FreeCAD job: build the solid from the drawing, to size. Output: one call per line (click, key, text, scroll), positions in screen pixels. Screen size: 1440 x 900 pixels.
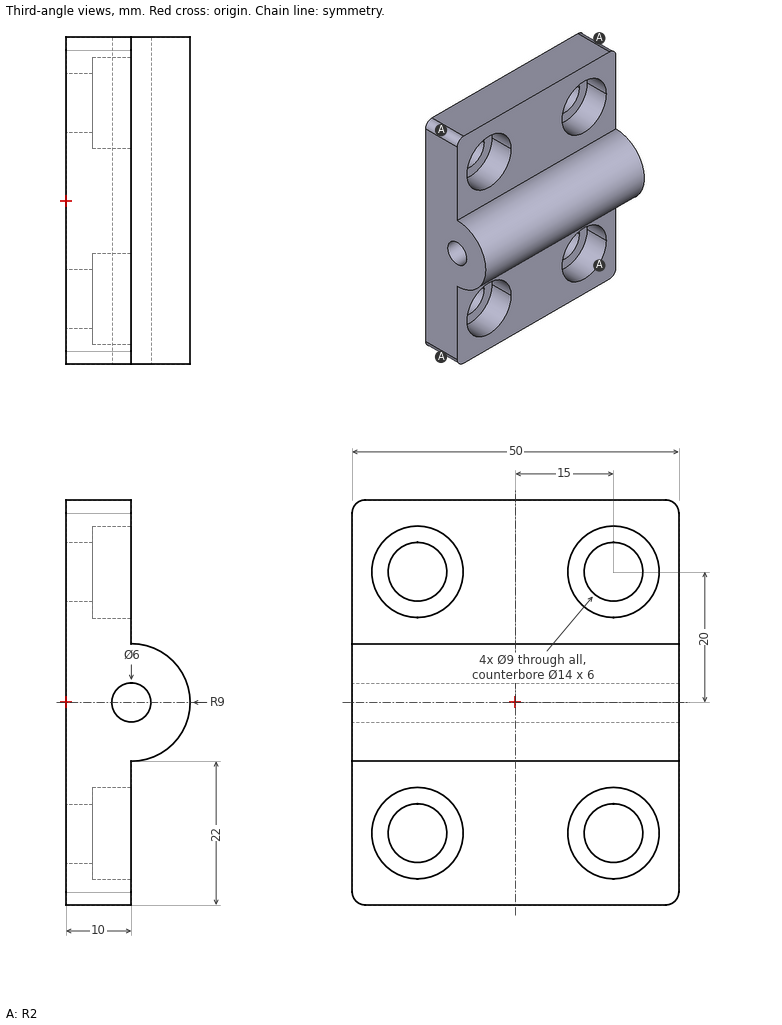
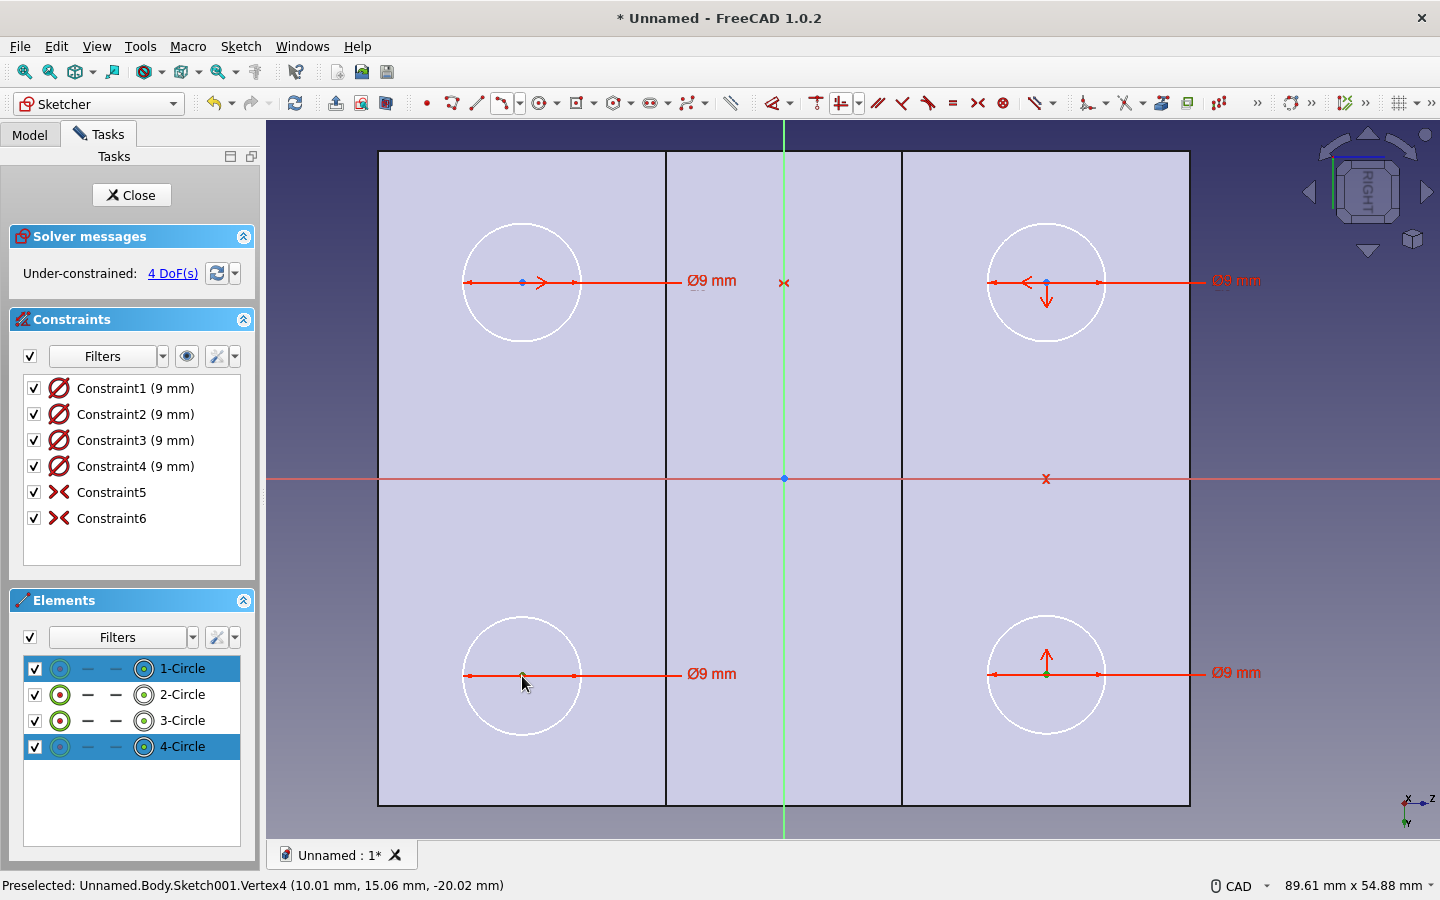
click(784, 764)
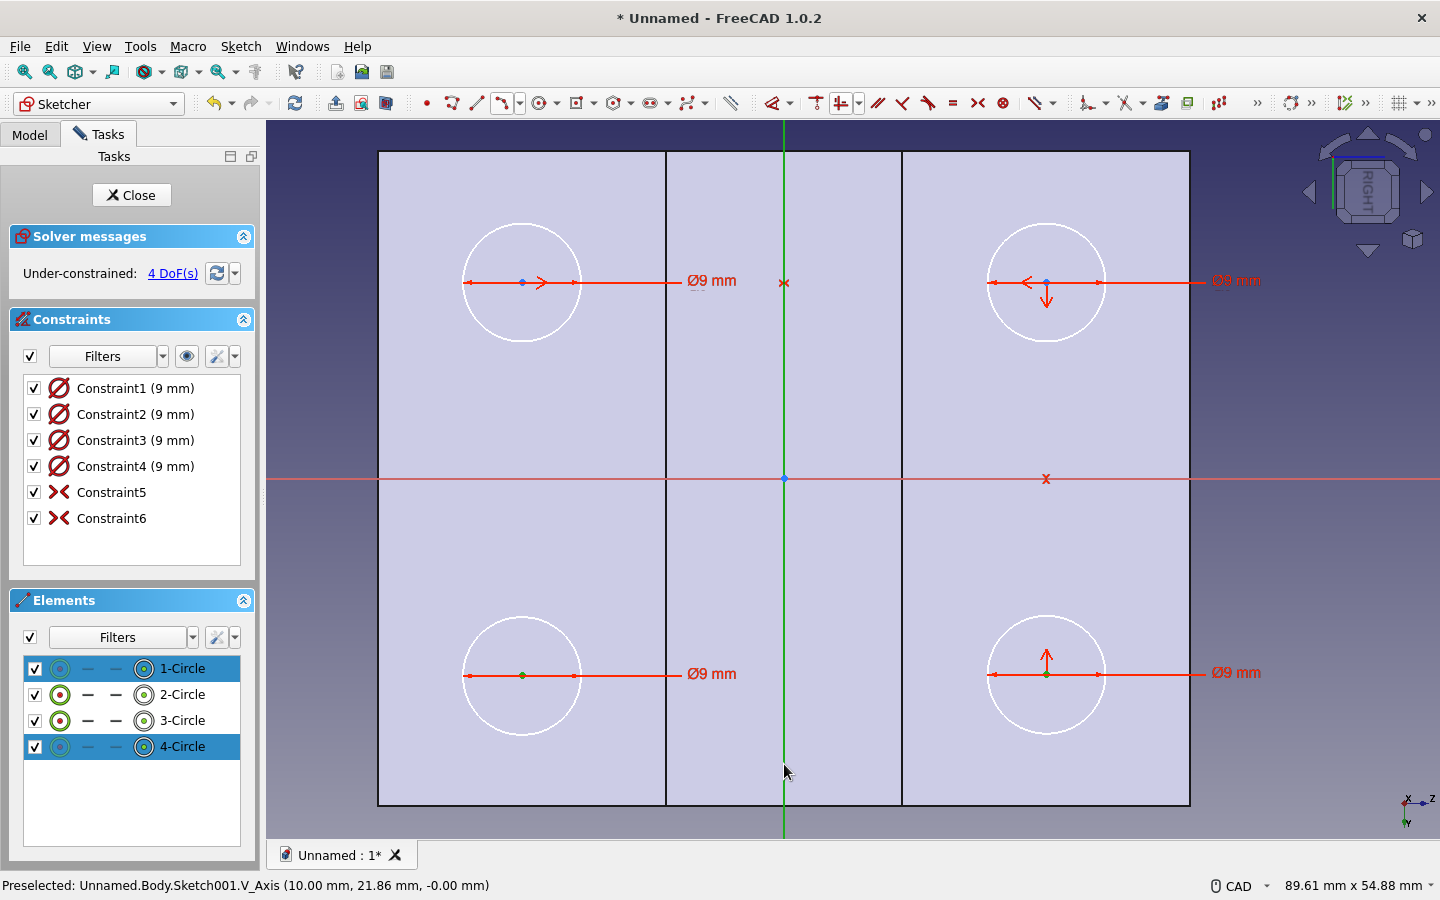
click(978, 104)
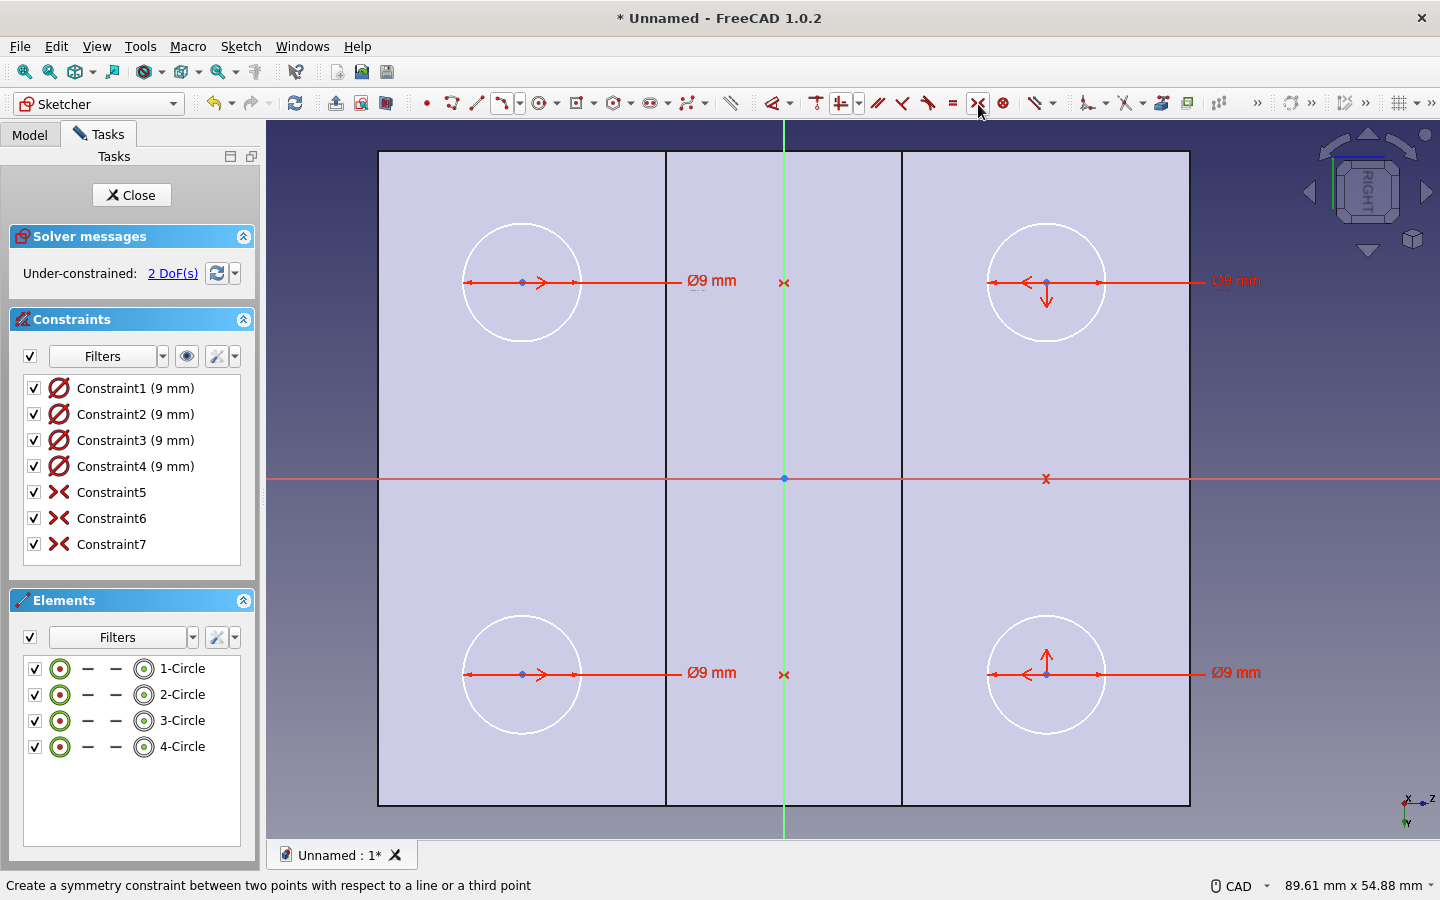
click(772, 104)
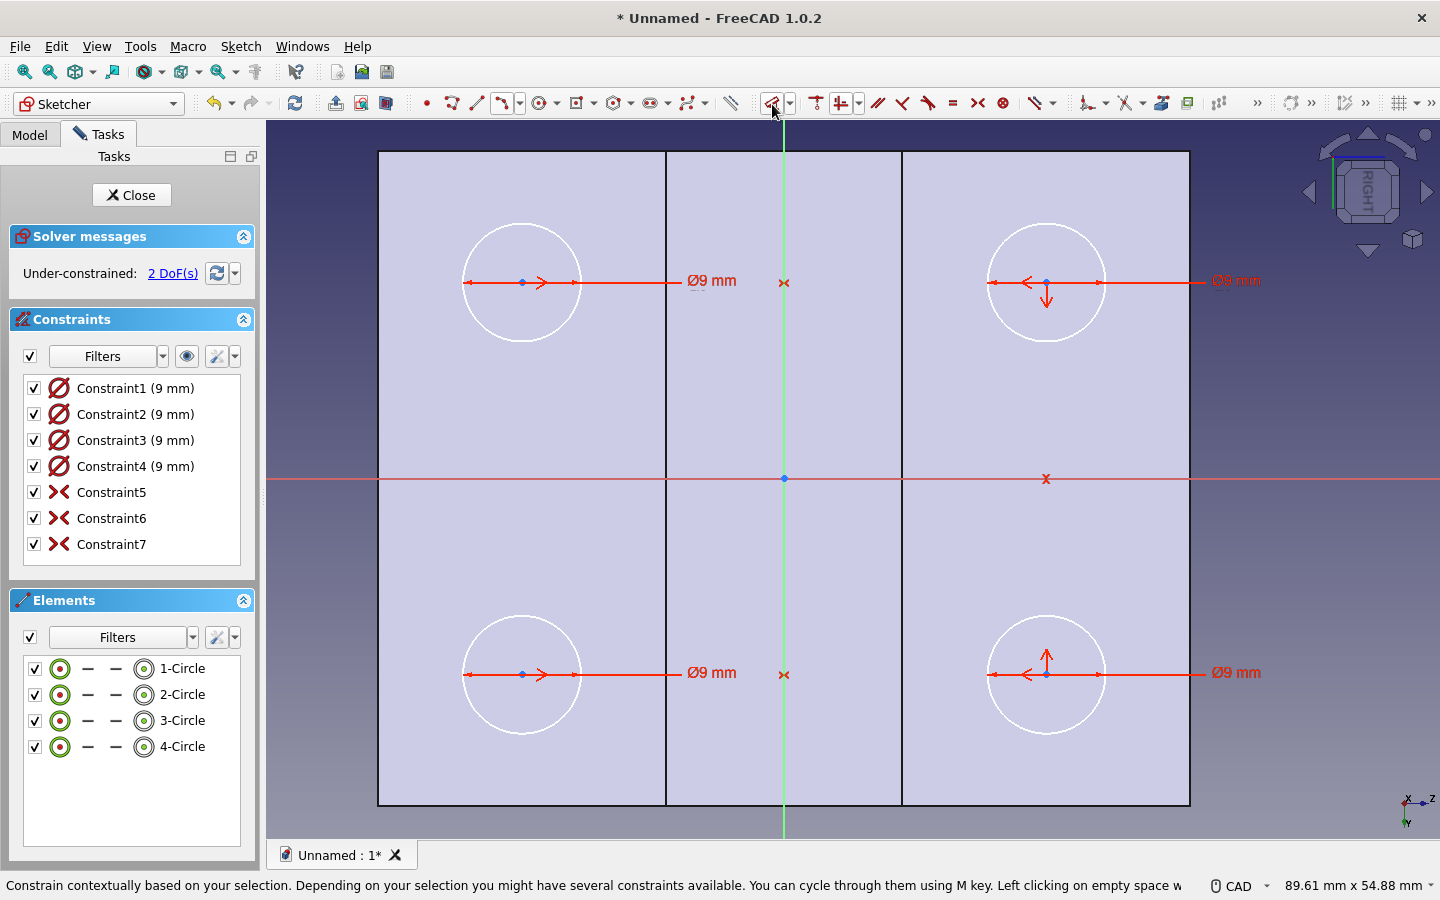
click(1047, 675)
click(915, 709)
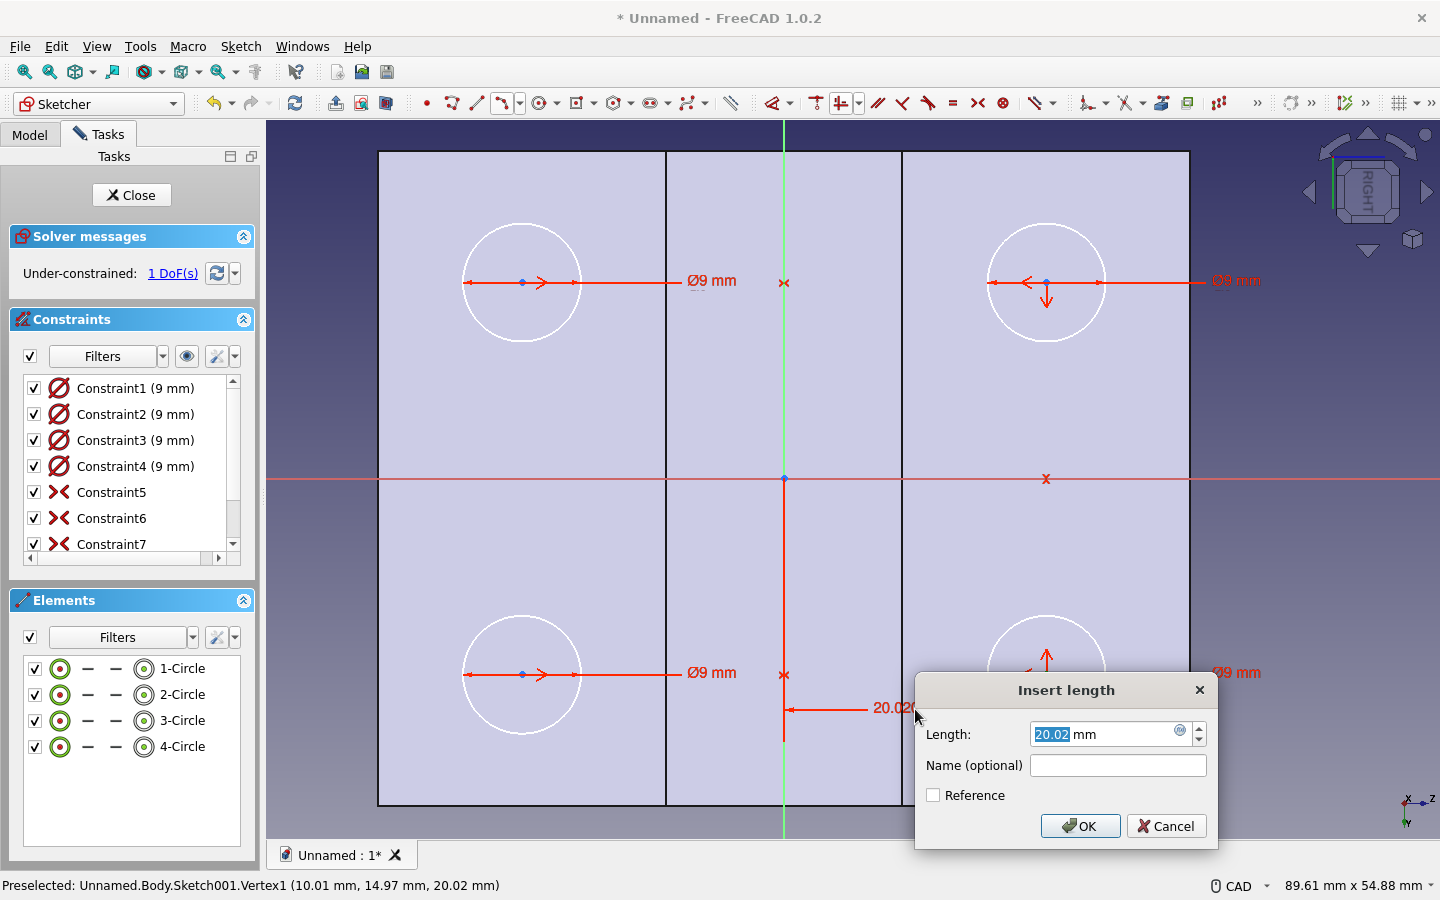
text(20)
key(Return)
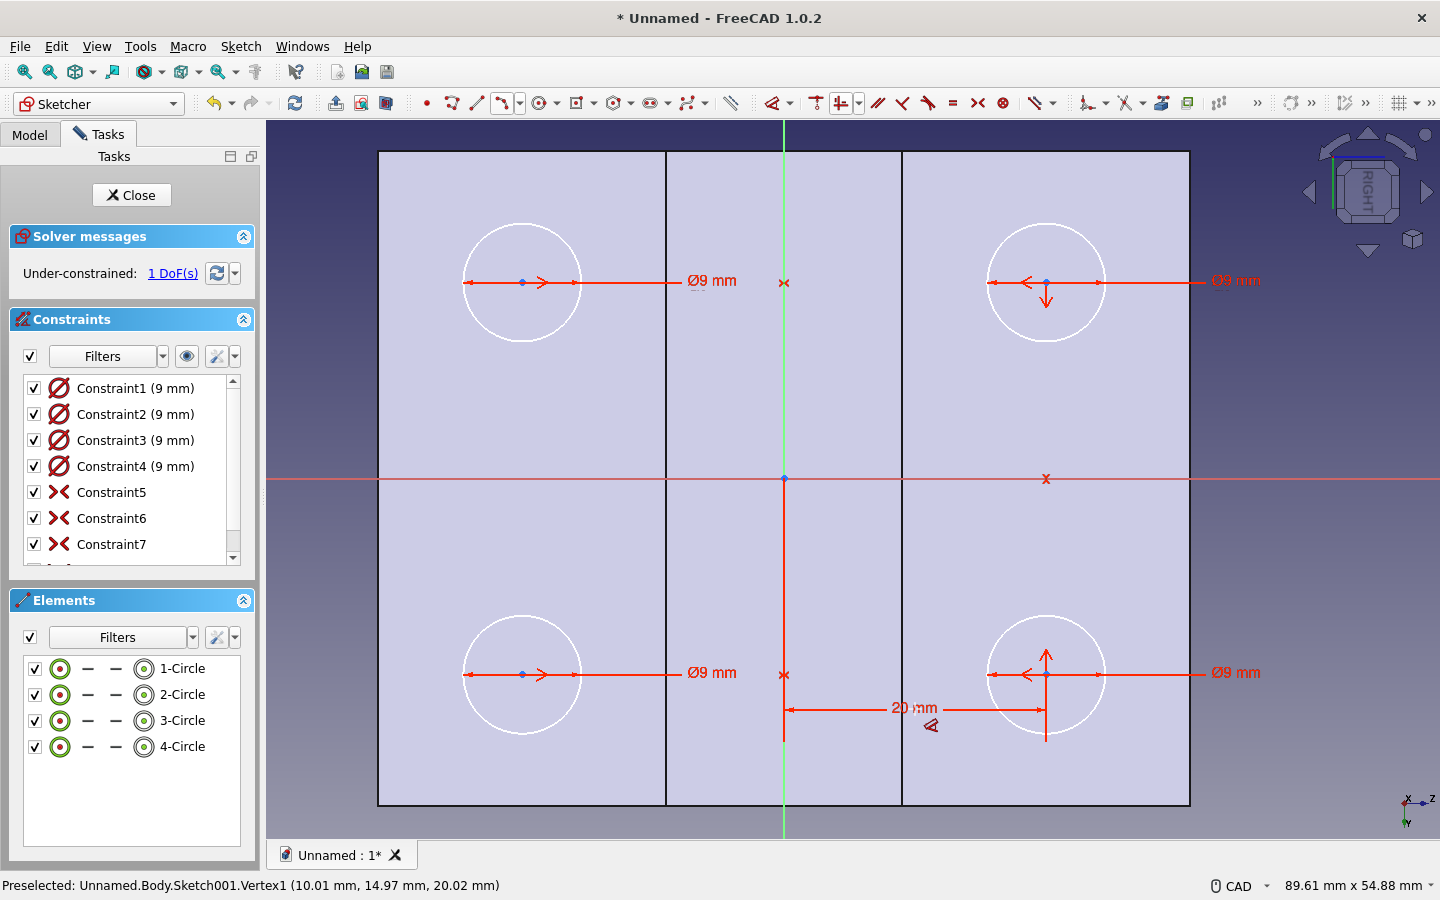
click(1046, 675)
click(1080, 577)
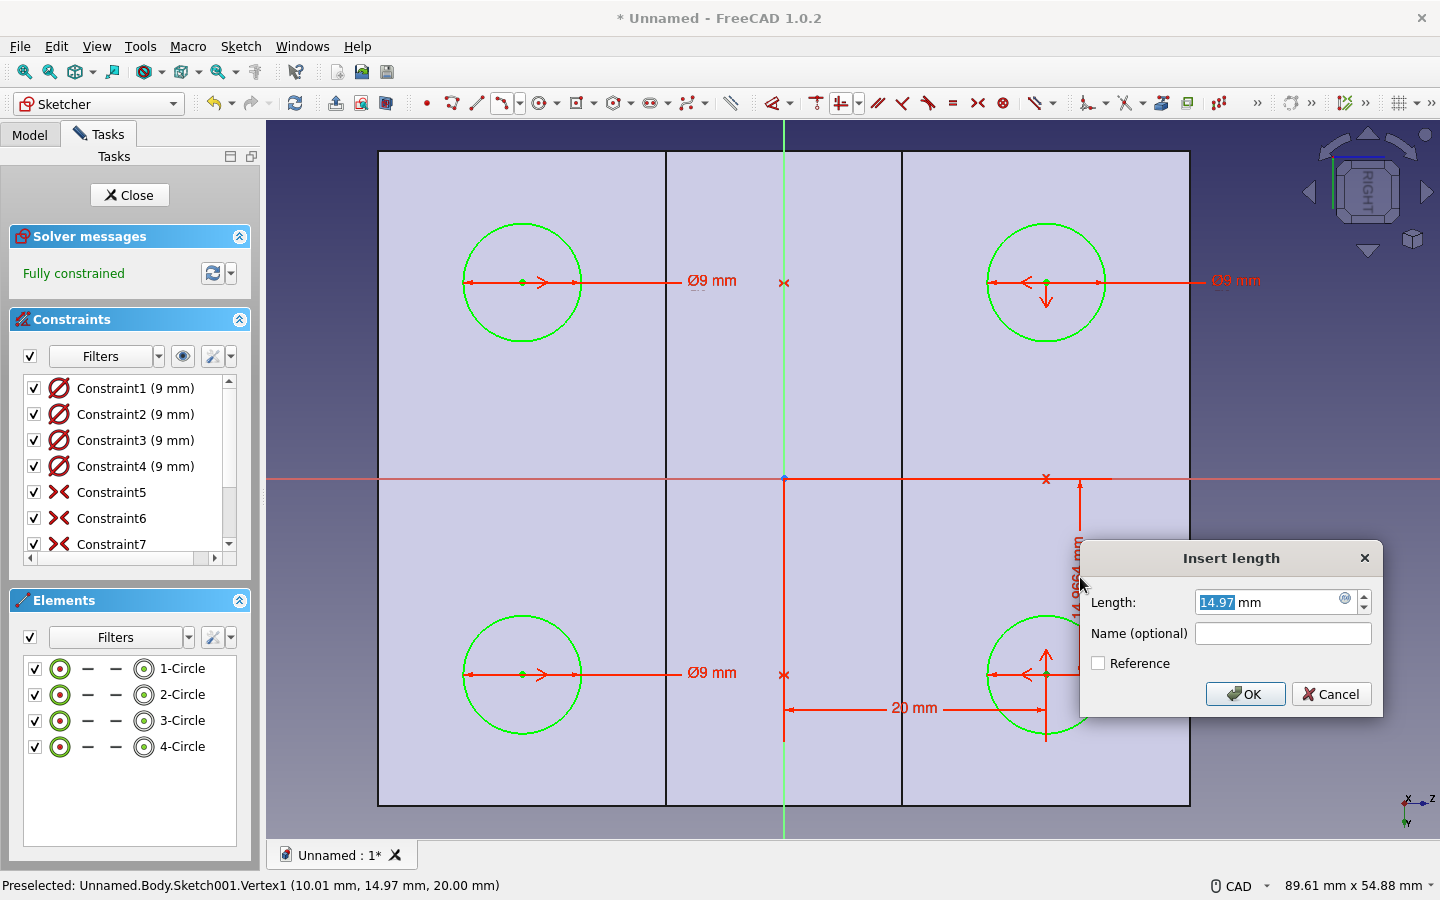
text(15)
key(Return)
key(Escape)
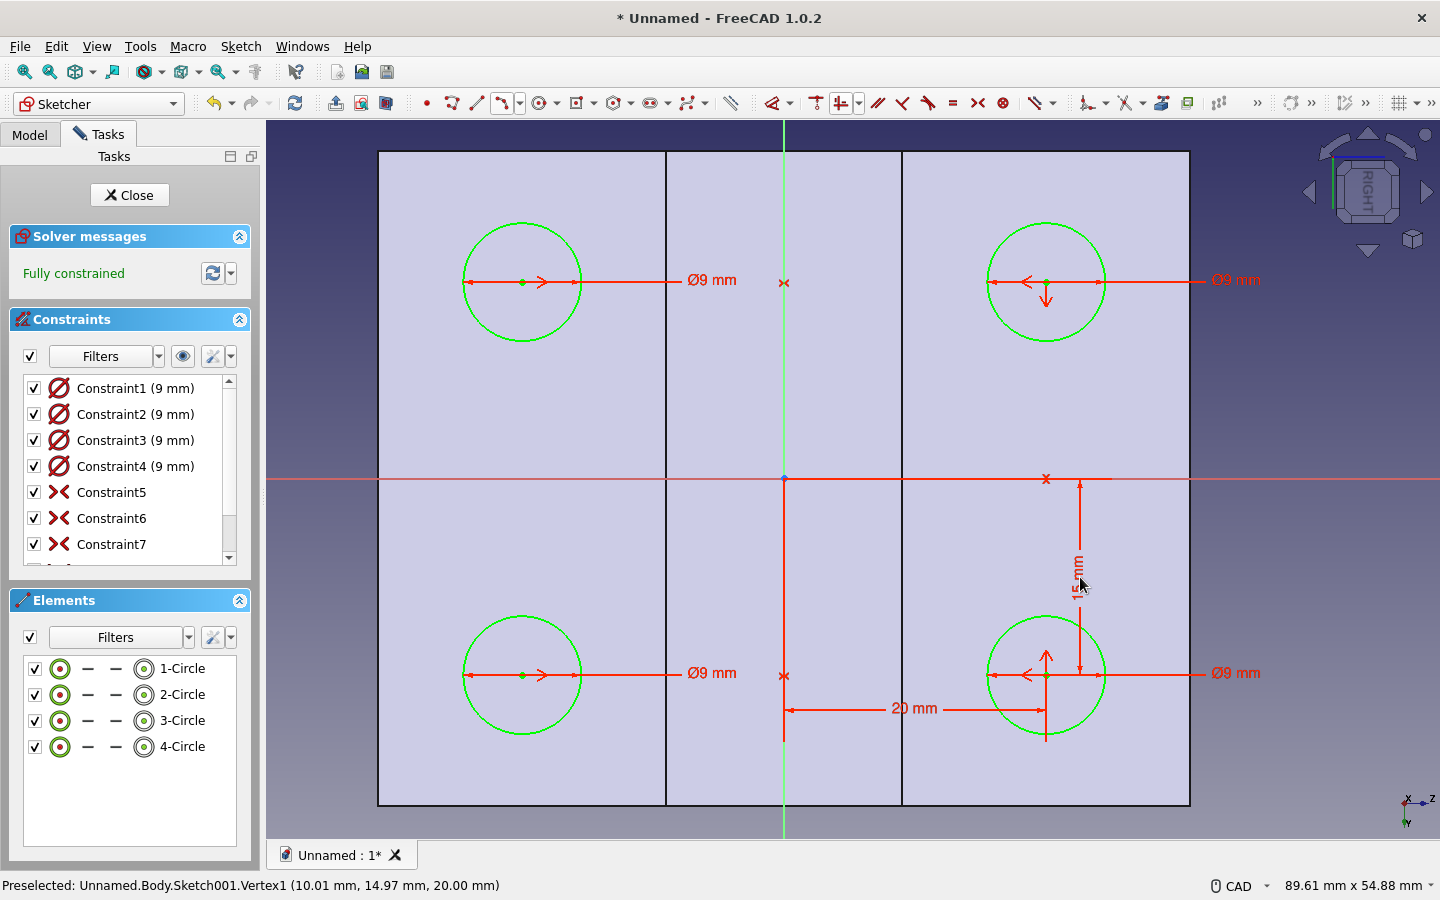
click(130, 195)